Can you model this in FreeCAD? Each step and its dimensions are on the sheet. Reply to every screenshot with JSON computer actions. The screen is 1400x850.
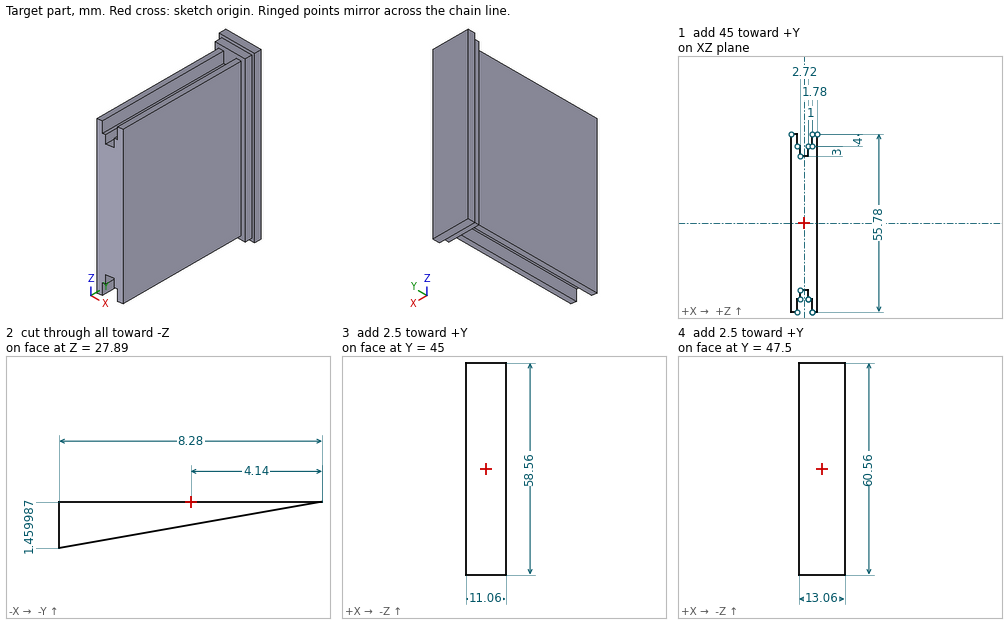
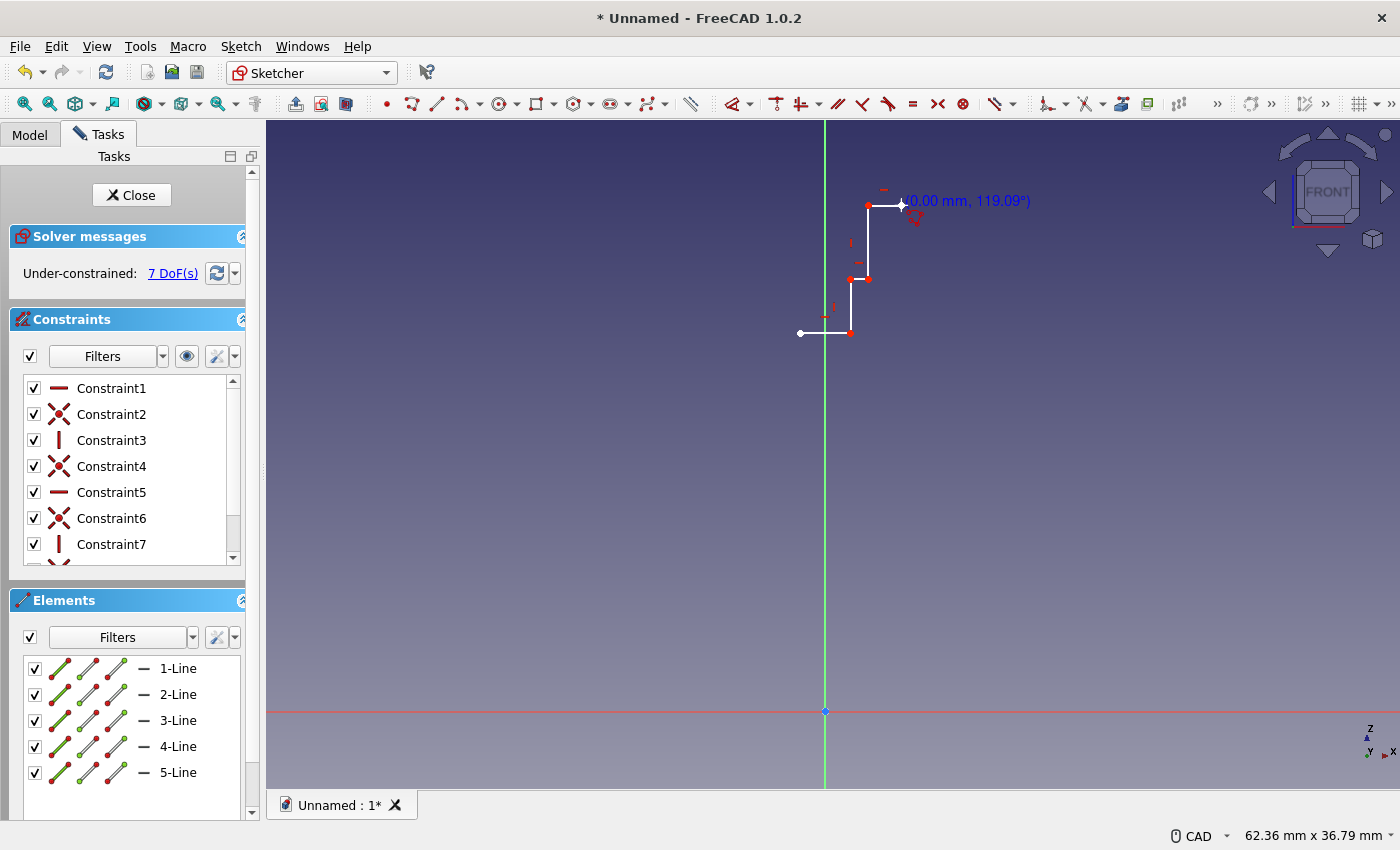
{"action": "scroll", "coordinate": [715, 244], "scroll_direction": "down", "scroll_amount": 4}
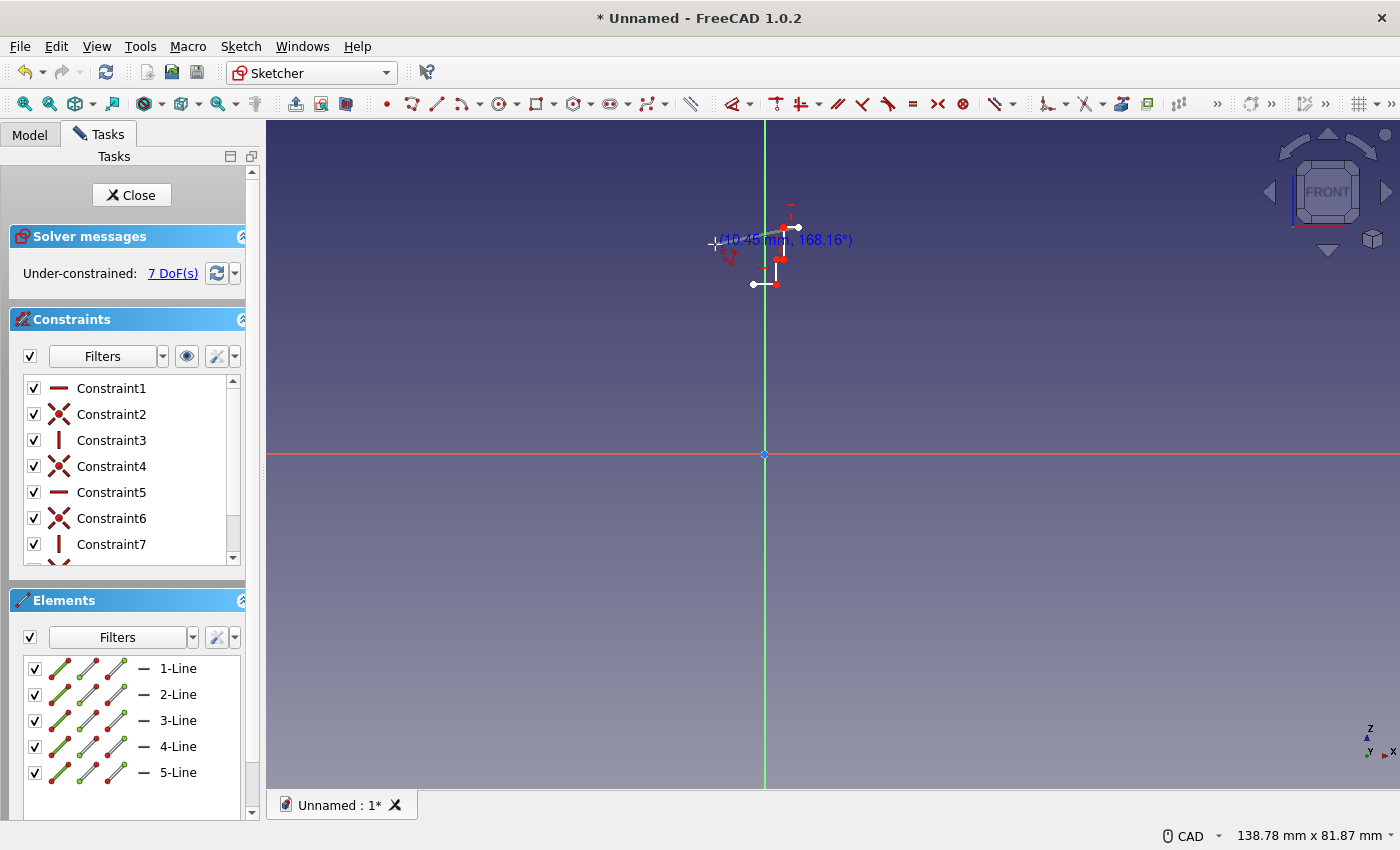
{"action": "left_click", "coordinate": [799, 682]}
{"action": "left_click", "coordinate": [784, 682]}
{"action": "left_click", "coordinate": [784, 650]}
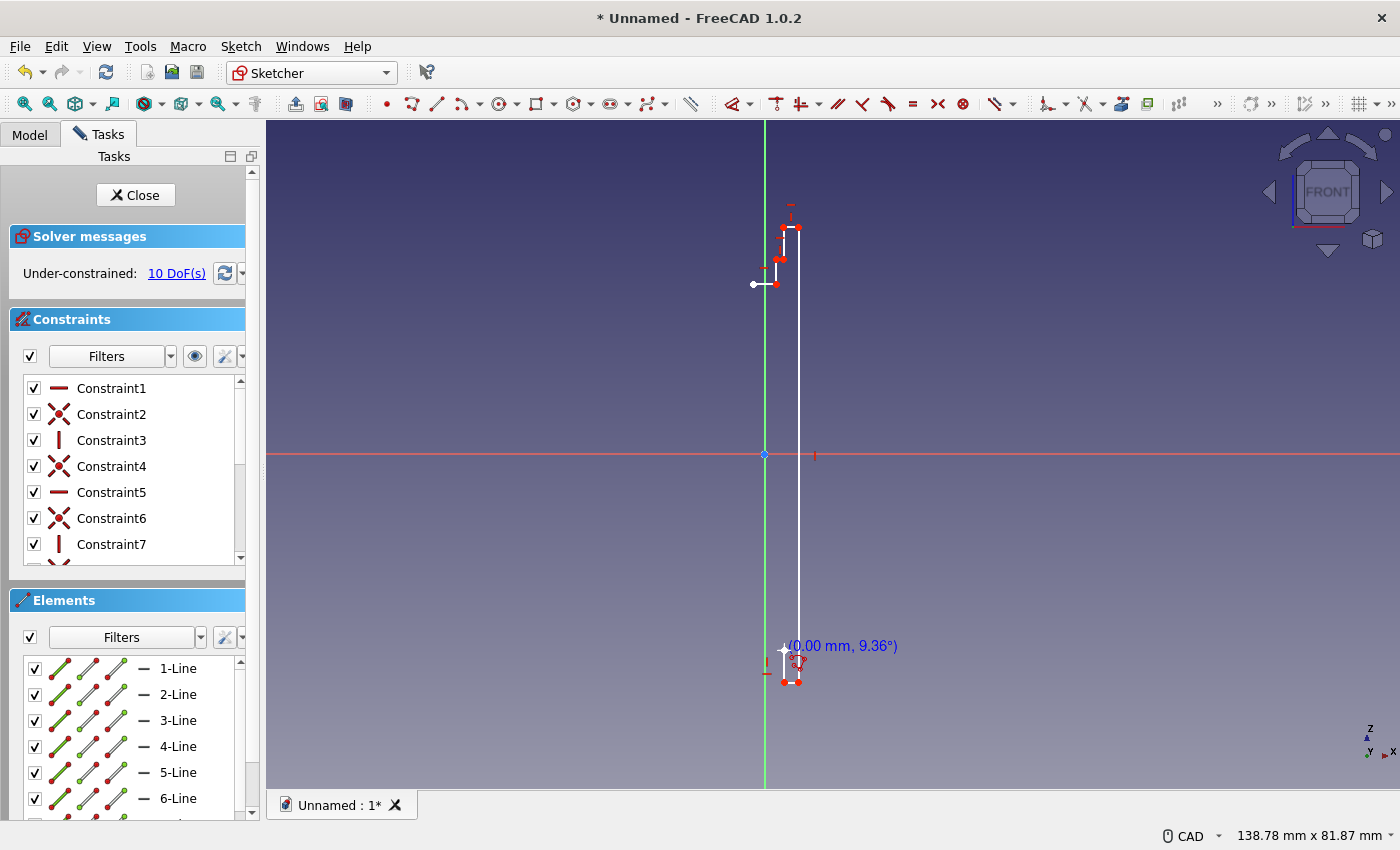
{"action": "scroll", "coordinate": [776, 650], "scroll_direction": "up", "scroll_amount": 4}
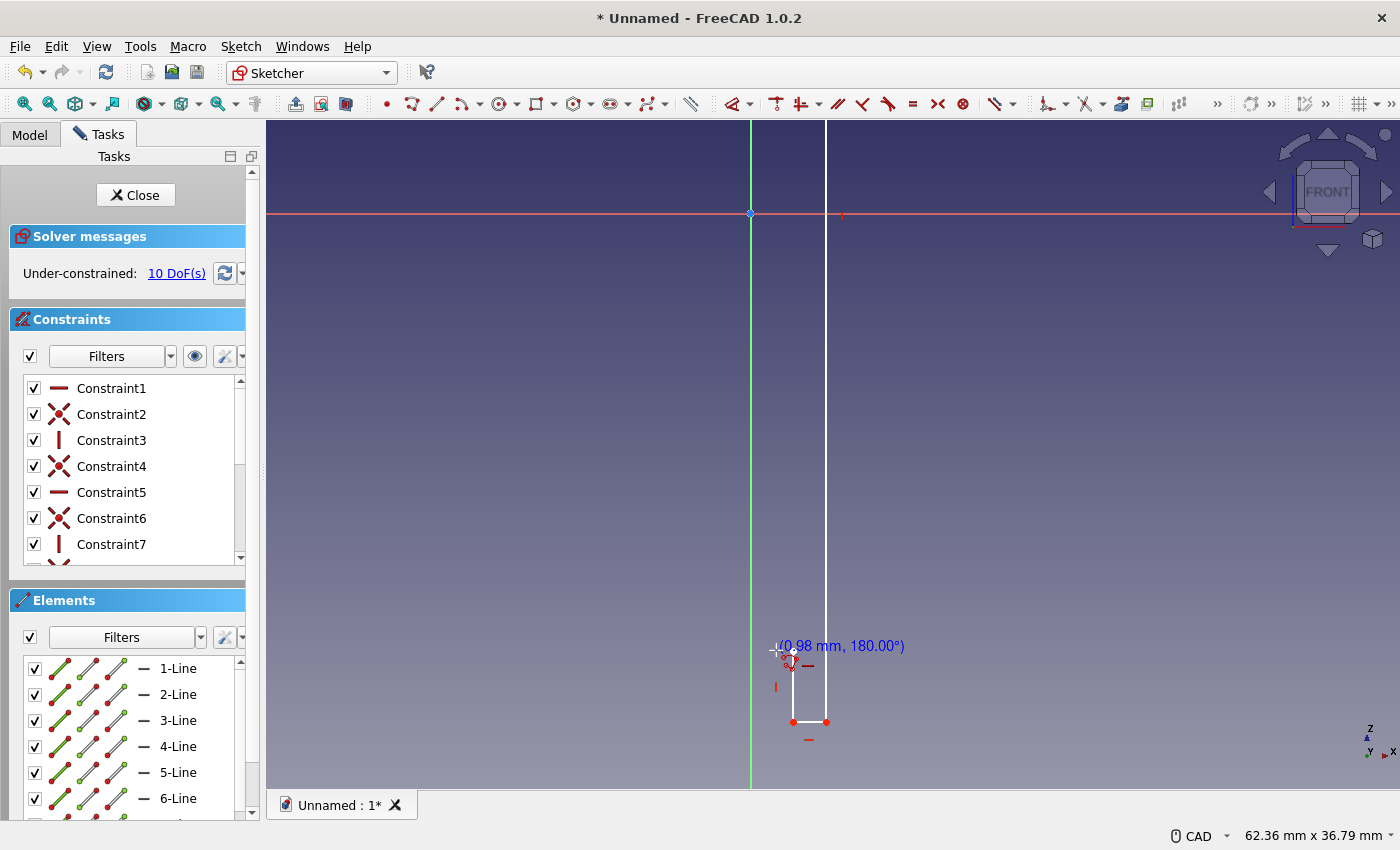
{"action": "left_click", "coordinate": [775, 649]}
{"action": "left_click", "coordinate": [775, 594]}
{"action": "left_click", "coordinate": [726, 594]}
{"action": "left_click", "coordinate": [726, 648]}
{"action": "left_click", "coordinate": [708, 648]}
{"action": "left_click", "coordinate": [708, 721]}
{"action": "left_click", "coordinate": [675, 721]}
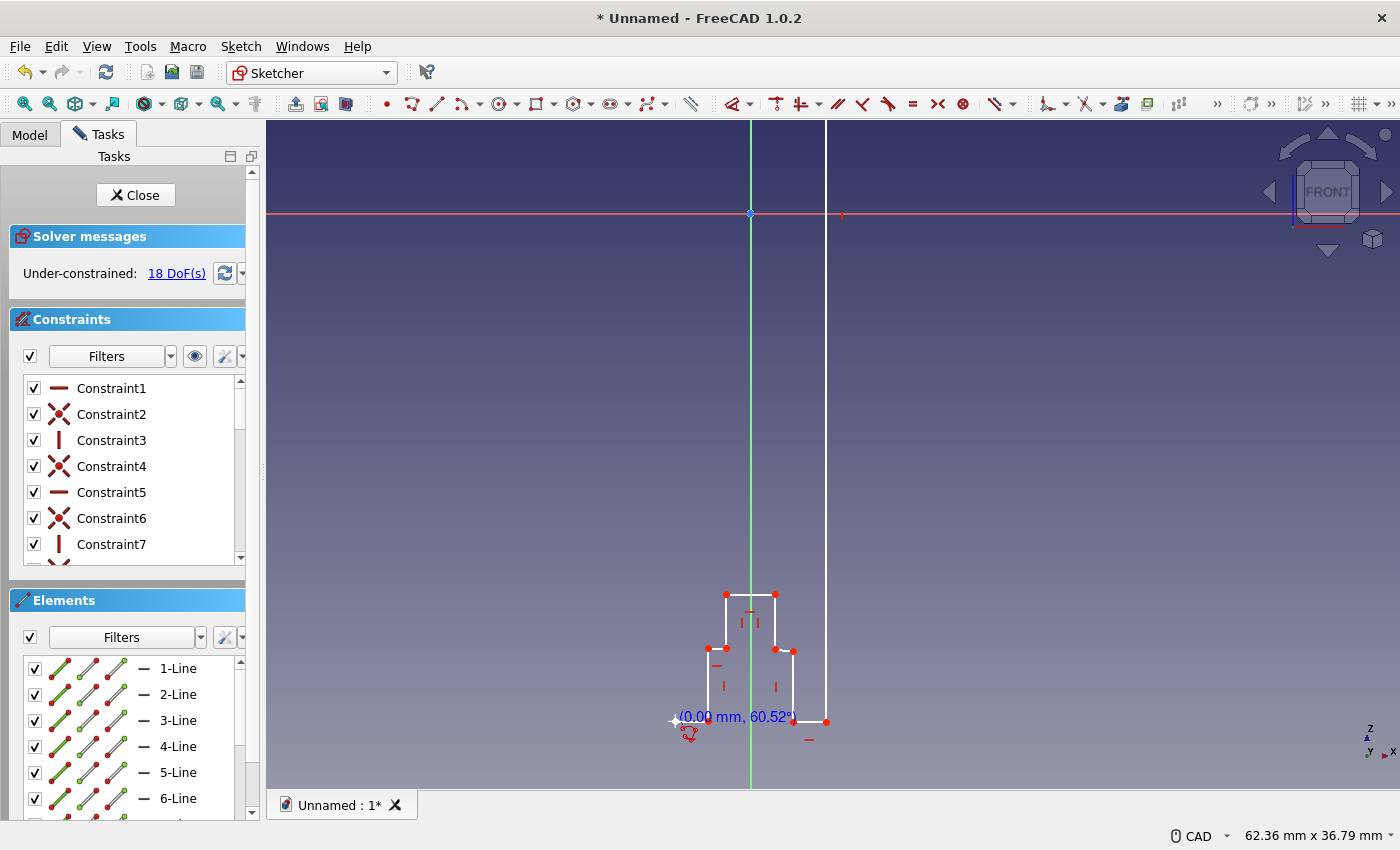
{"action": "scroll", "coordinate": [776, 651], "scroll_direction": "down", "scroll_amount": 4}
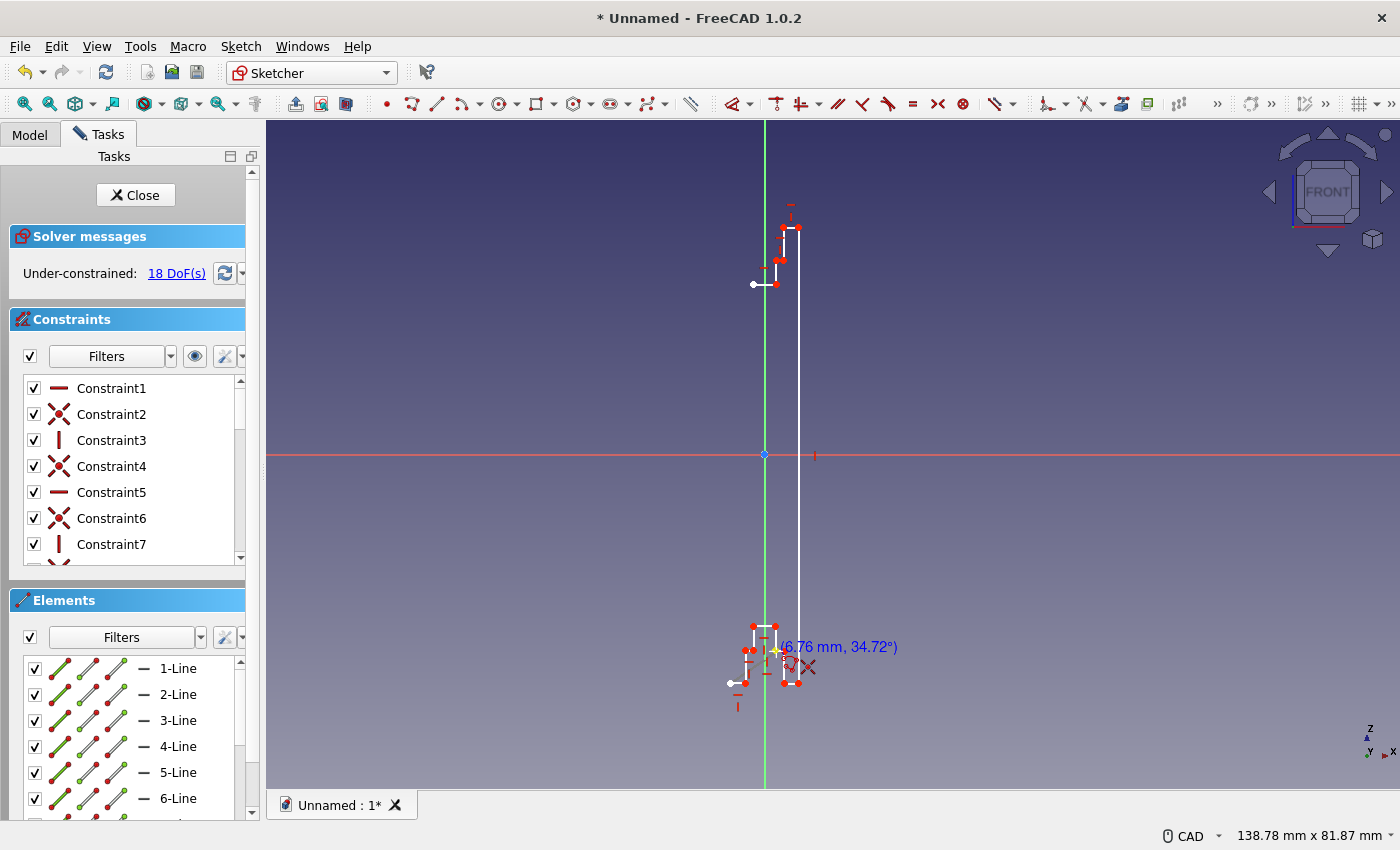
{"action": "left_click", "coordinate": [731, 227]}
{"action": "left_click", "coordinate": [746, 227]}
{"action": "left_click", "coordinate": [746, 260]}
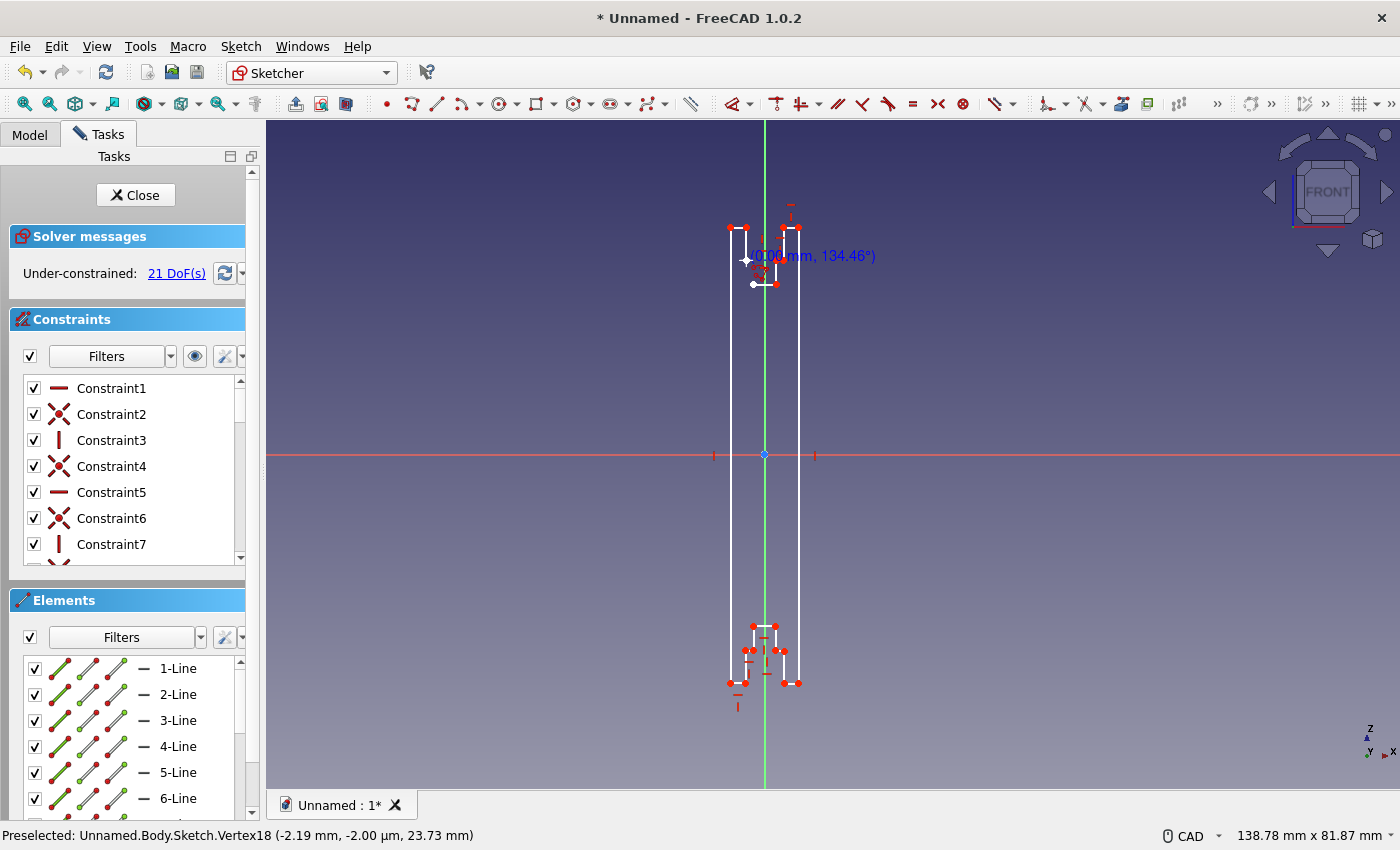
{"action": "scroll", "coordinate": [754, 260], "scroll_direction": "up", "scroll_amount": 4}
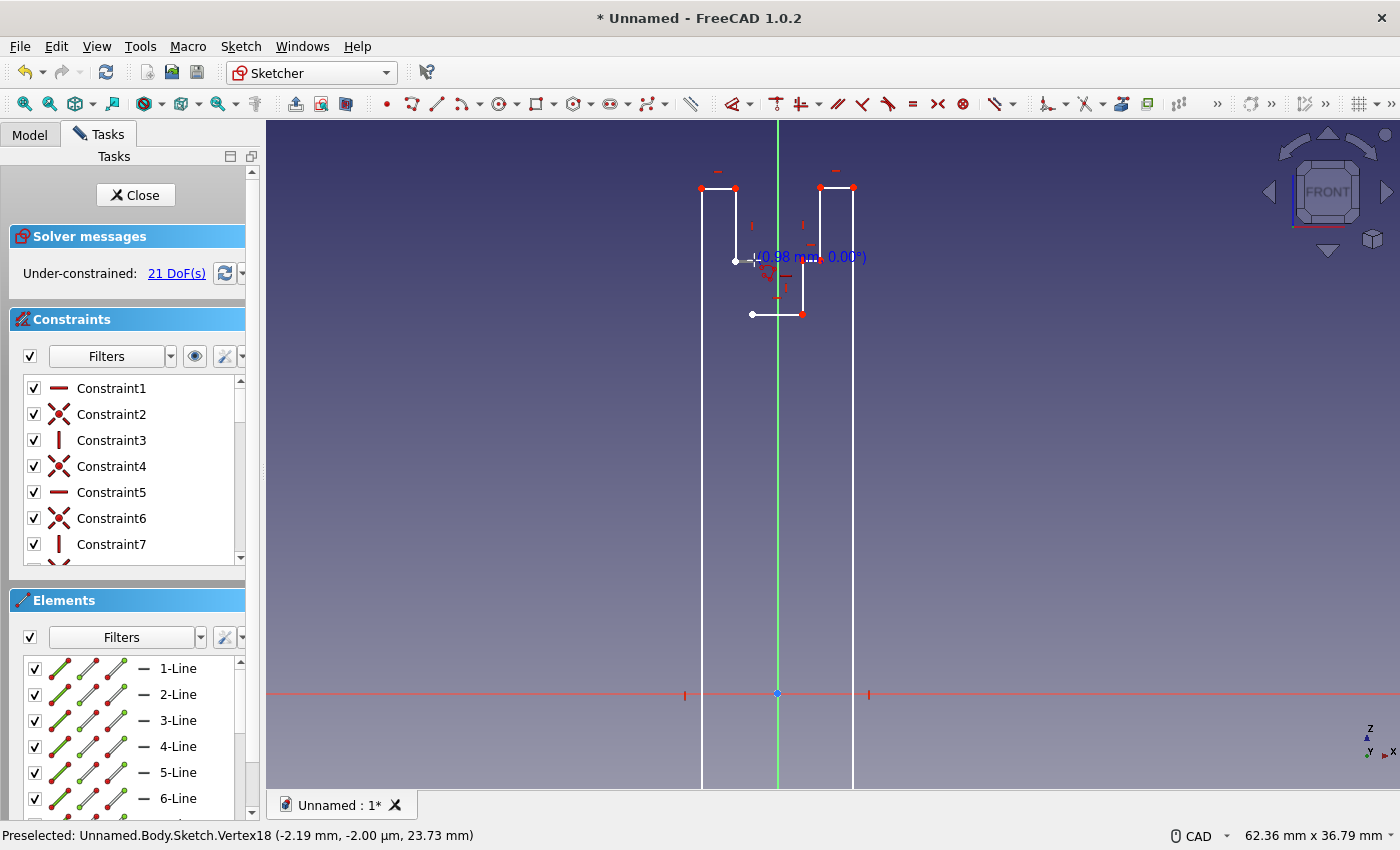
{"action": "left_click", "coordinate": [753, 260]}
{"action": "left_click", "coordinate": [752, 315]}
{"action": "key", "text": "Escape"}
{"action": "key", "text": "Escape"}